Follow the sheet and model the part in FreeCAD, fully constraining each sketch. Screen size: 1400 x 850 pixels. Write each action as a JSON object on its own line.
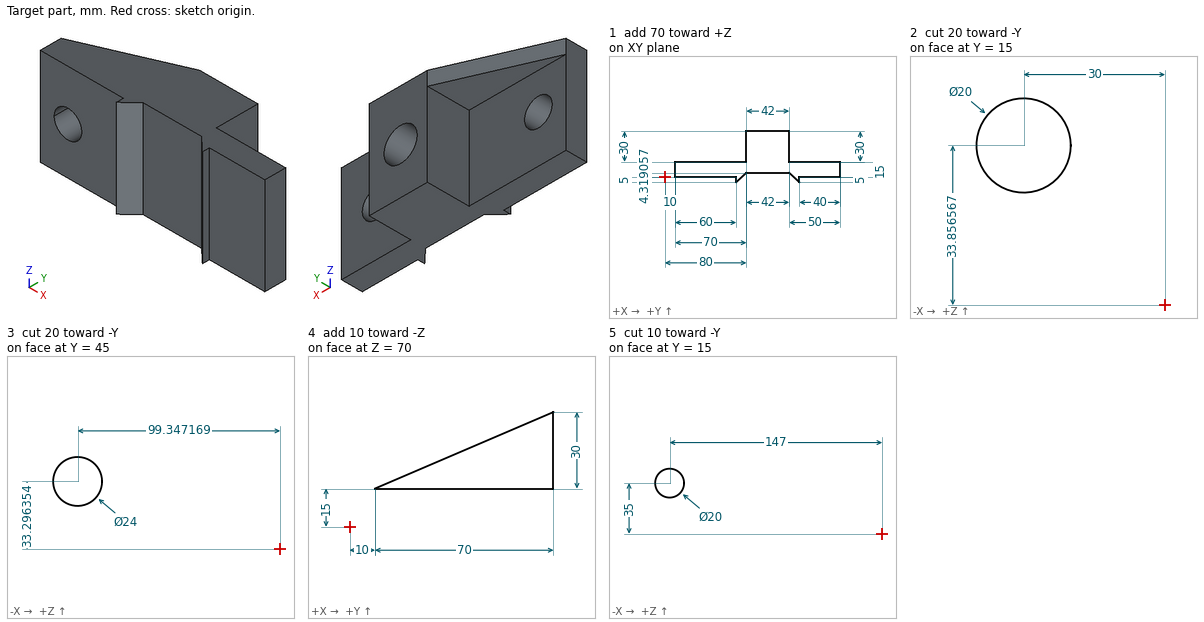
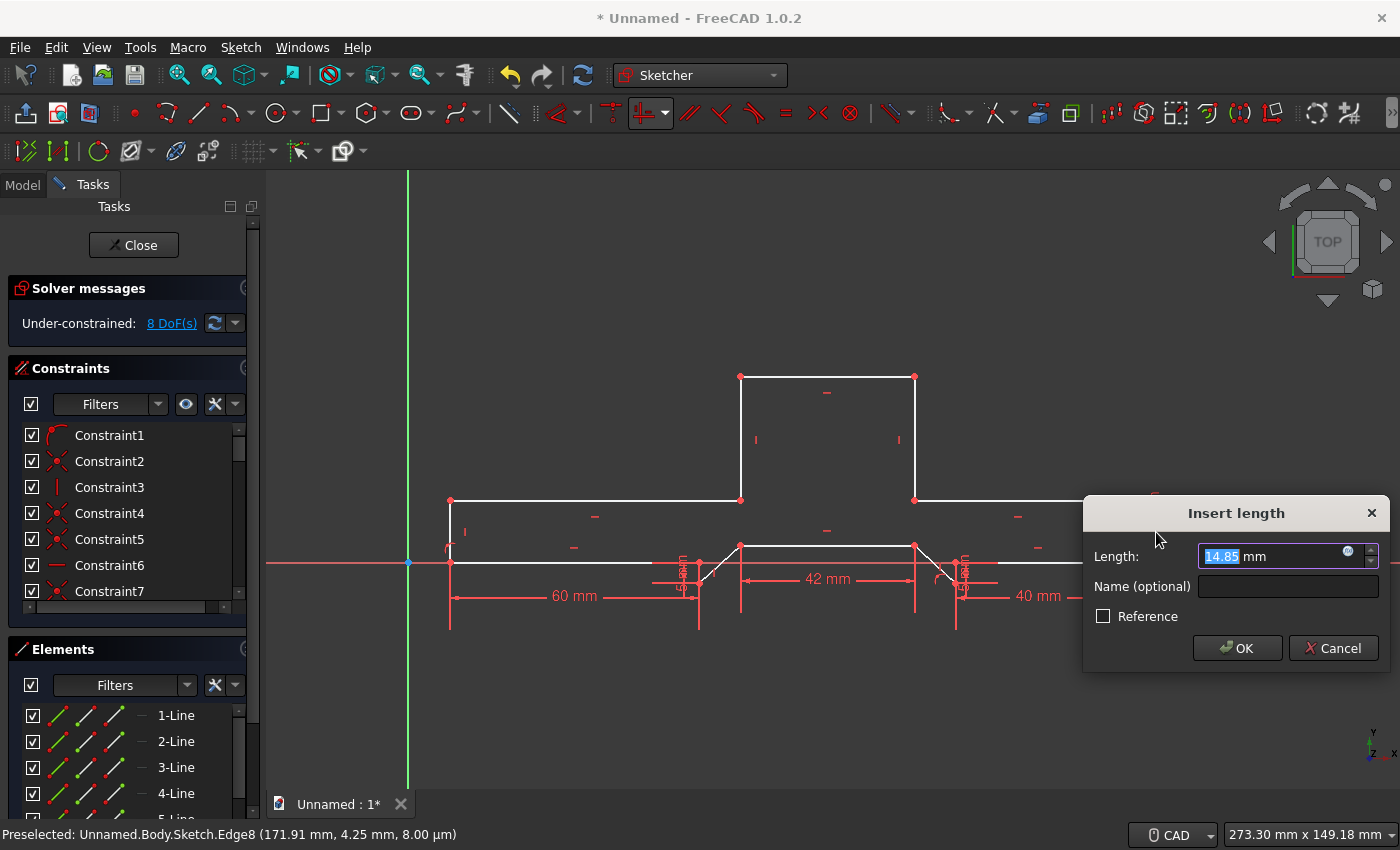
{"action": "type", "text": "15"}
{"action": "key", "text": "Return"}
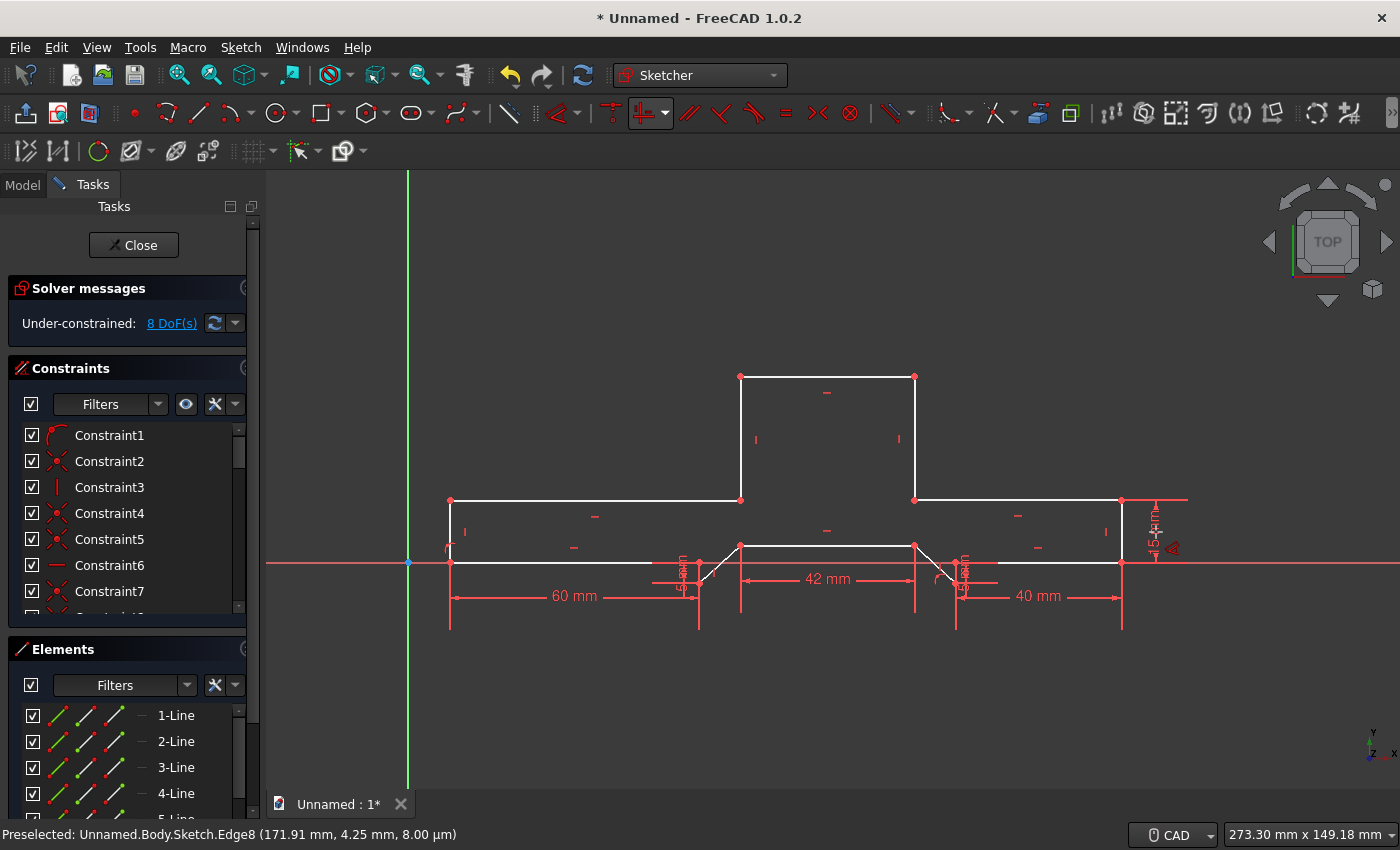
{"action": "left_click", "coordinate": [1060, 500]}
{"action": "left_click", "coordinate": [1018, 534]}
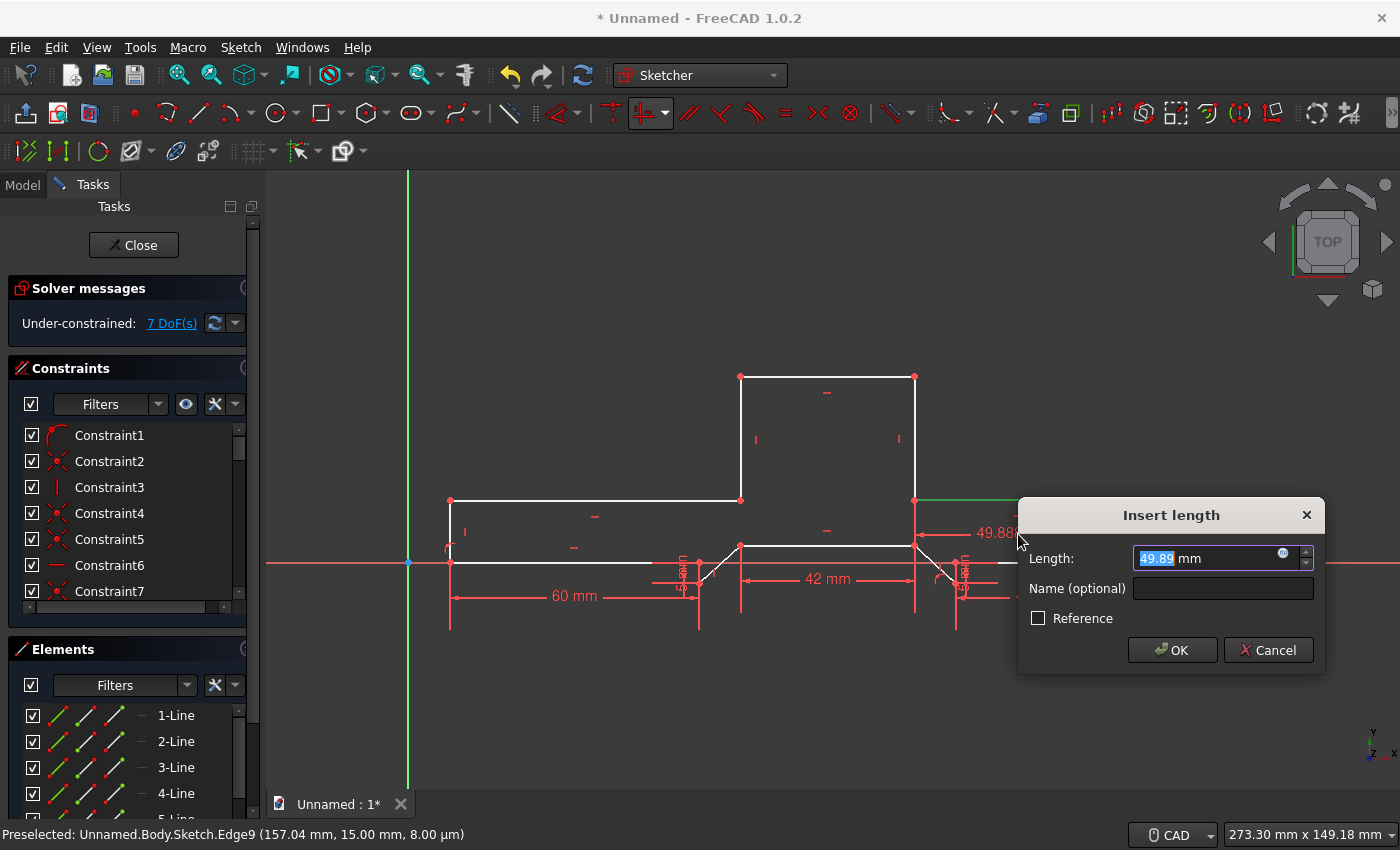
{"action": "type", "text": "50"}
{"action": "key", "text": "Return"}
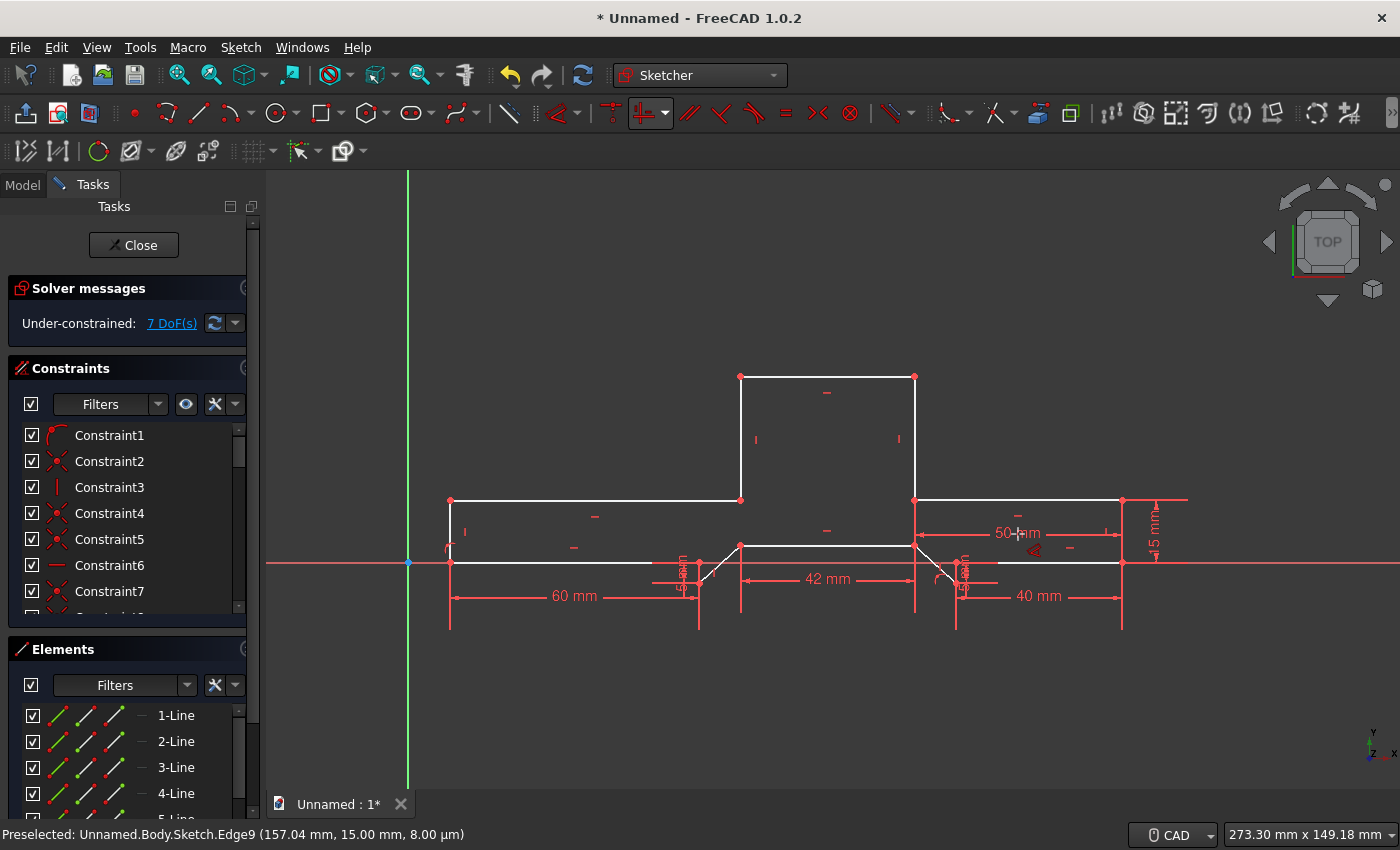
{"action": "left_click", "coordinate": [915, 463]}
{"action": "left_click", "coordinate": [949, 439]}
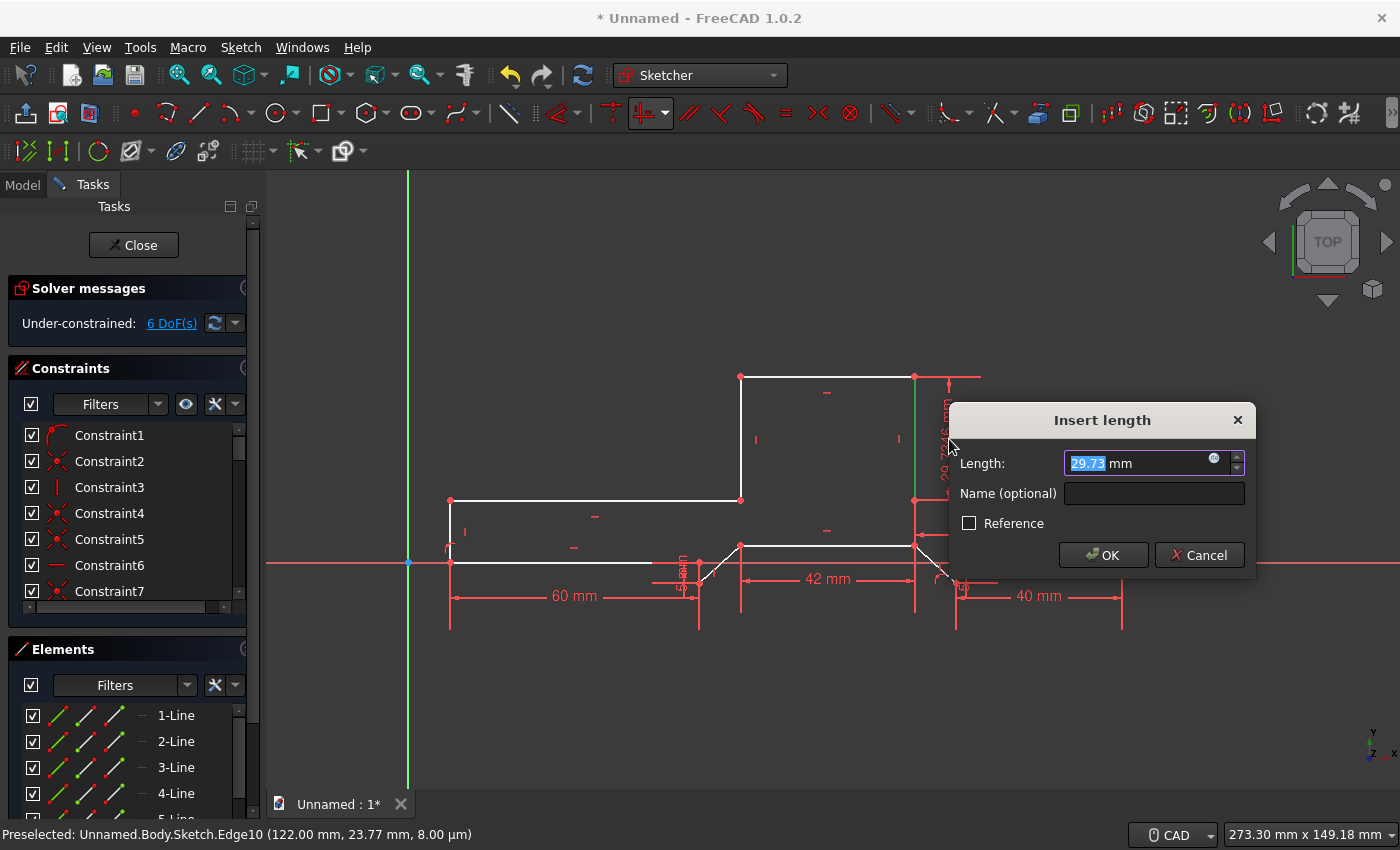
{"action": "type", "text": "30"}
{"action": "key", "text": "Return"}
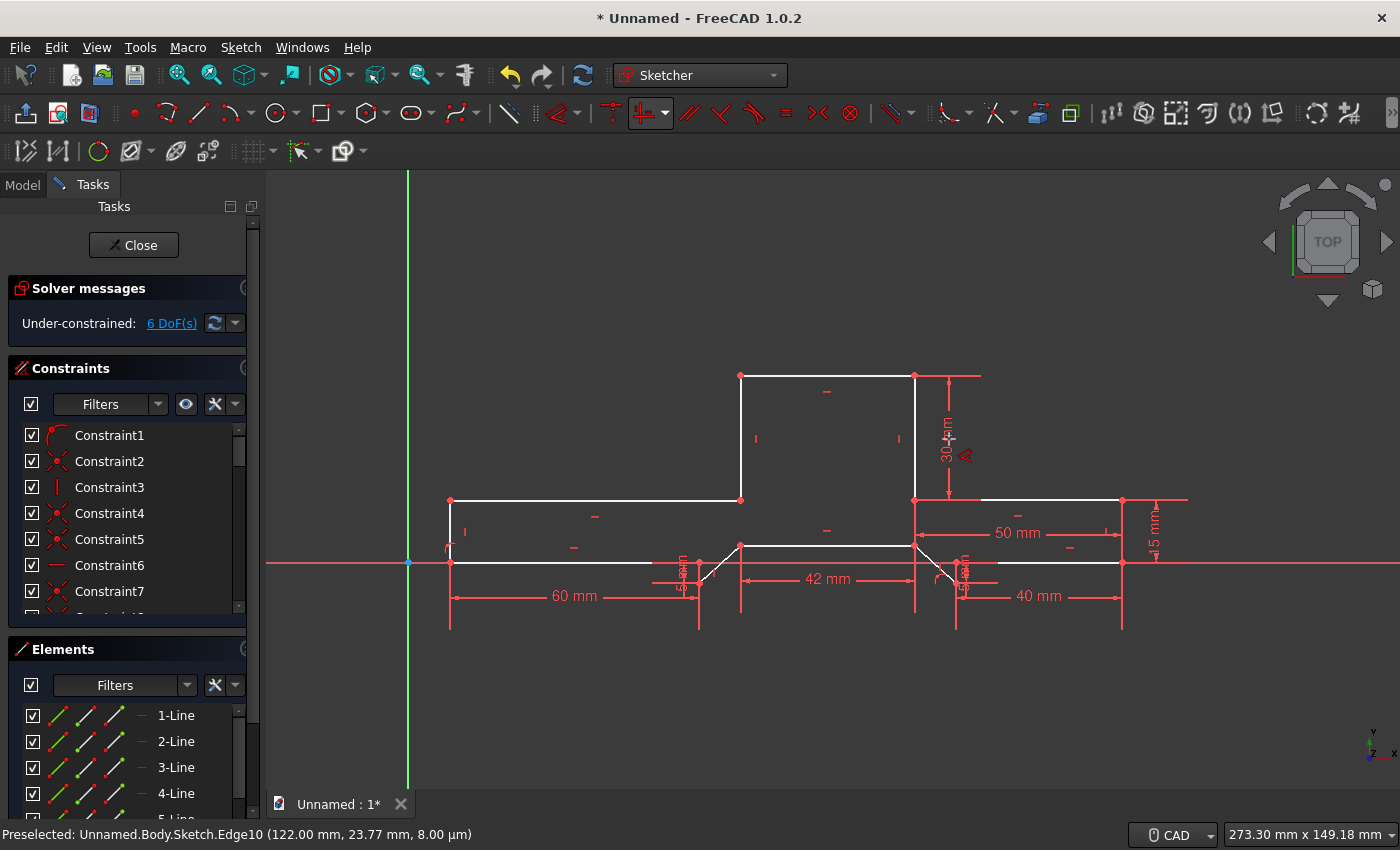
{"action": "left_click", "coordinate": [862, 376]}
{"action": "left_click", "coordinate": [828, 342]}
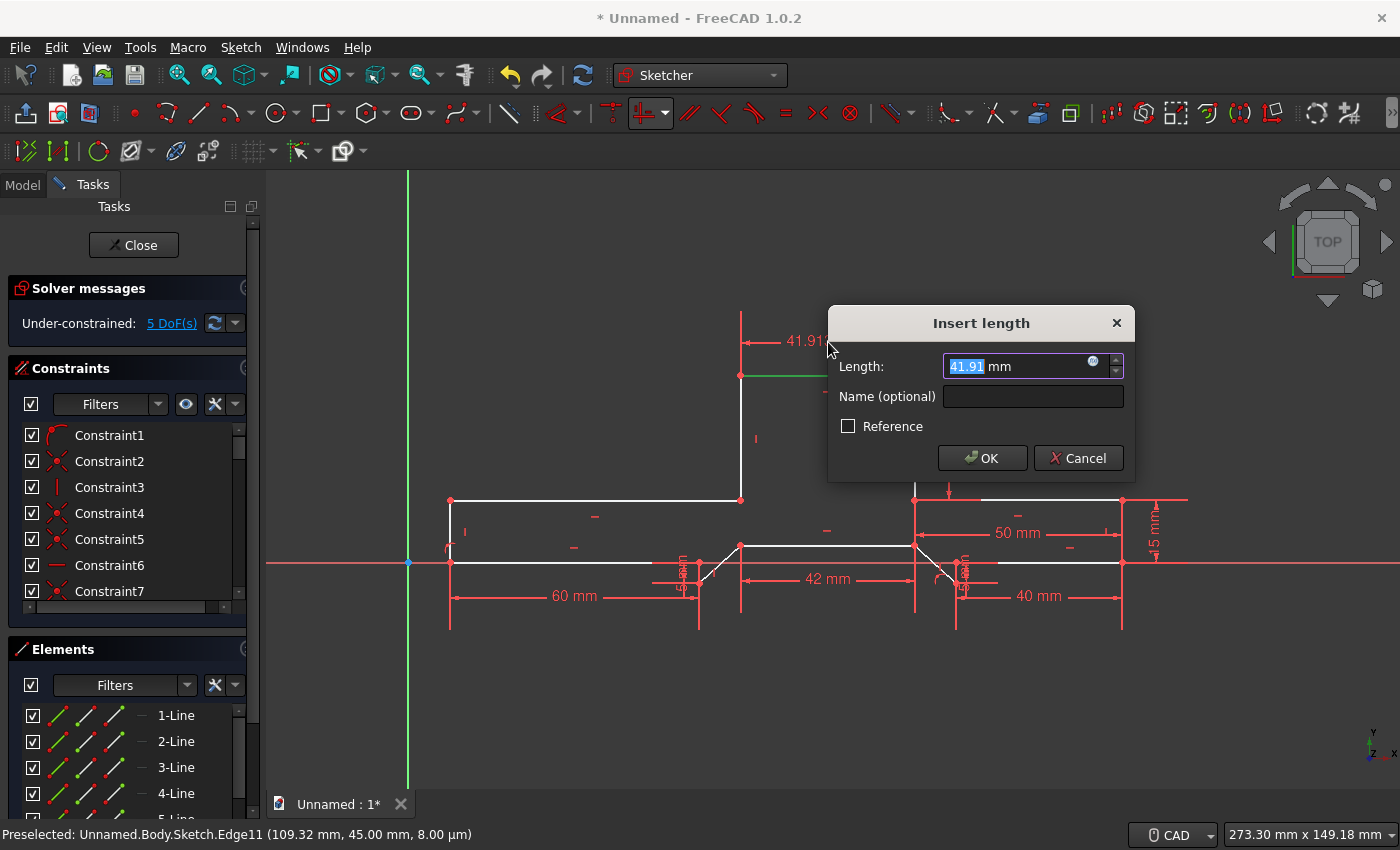
{"action": "type", "text": "42"}
{"action": "key", "text": "Return"}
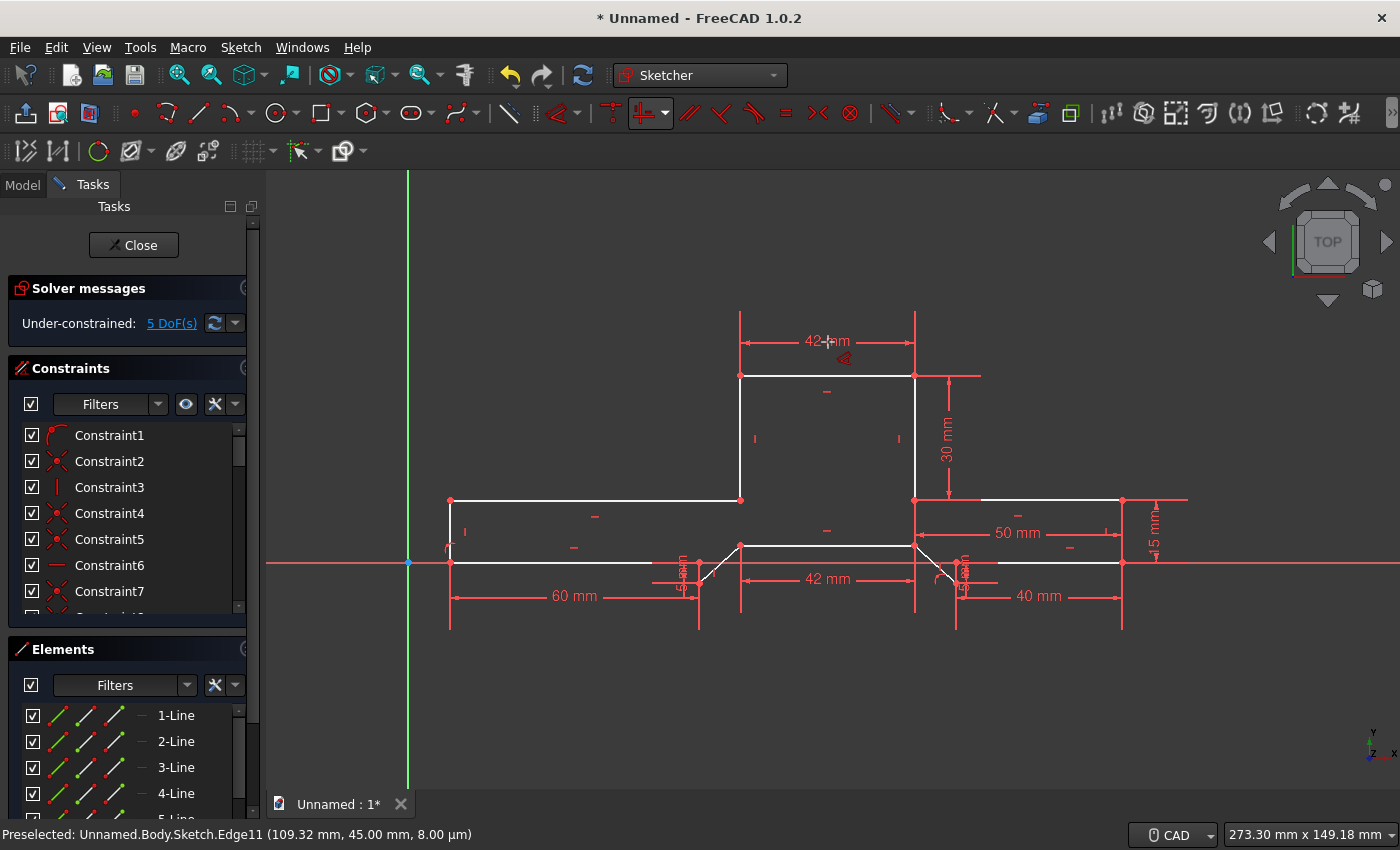
{"action": "left_click", "coordinate": [740, 413]}
{"action": "left_click", "coordinate": [706, 438]}